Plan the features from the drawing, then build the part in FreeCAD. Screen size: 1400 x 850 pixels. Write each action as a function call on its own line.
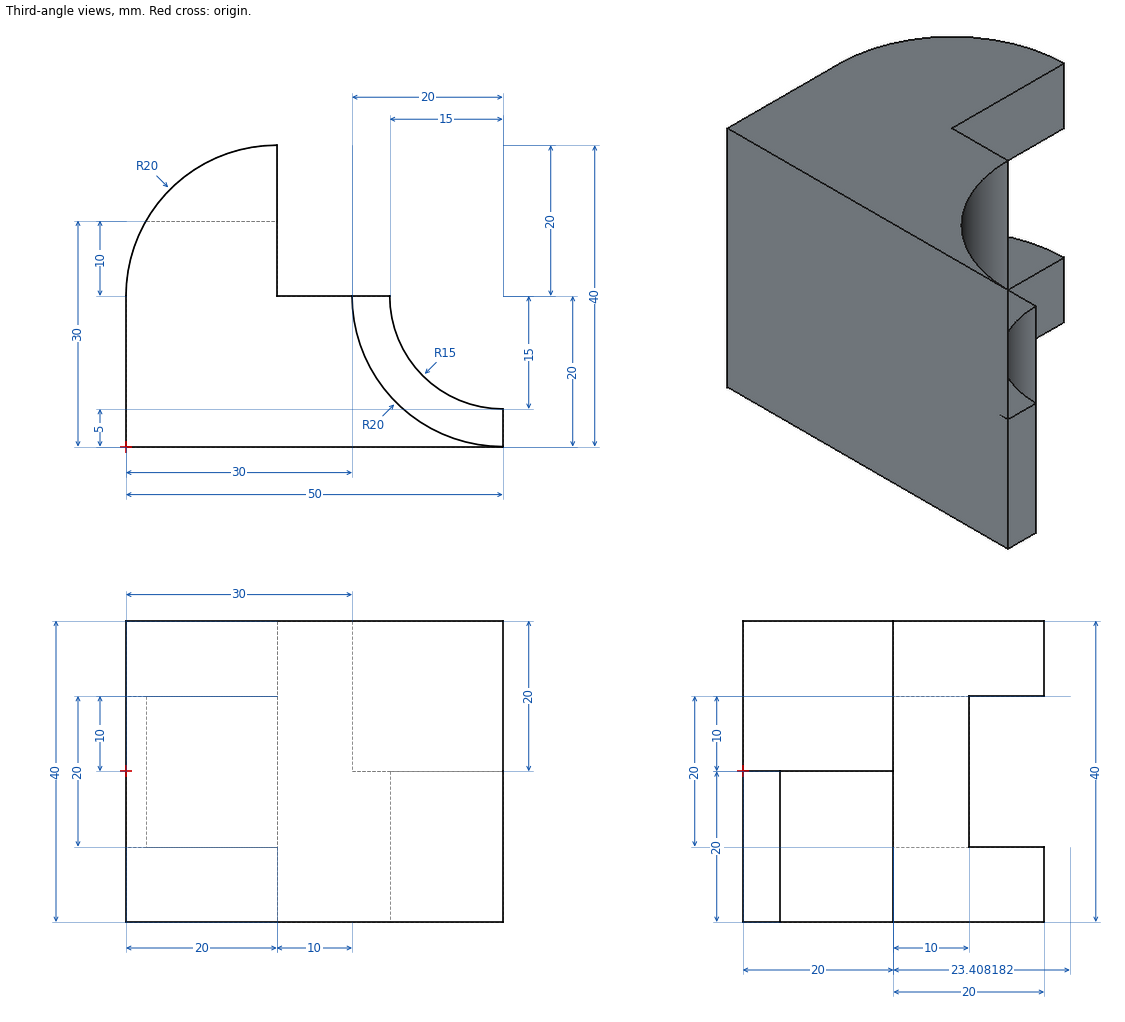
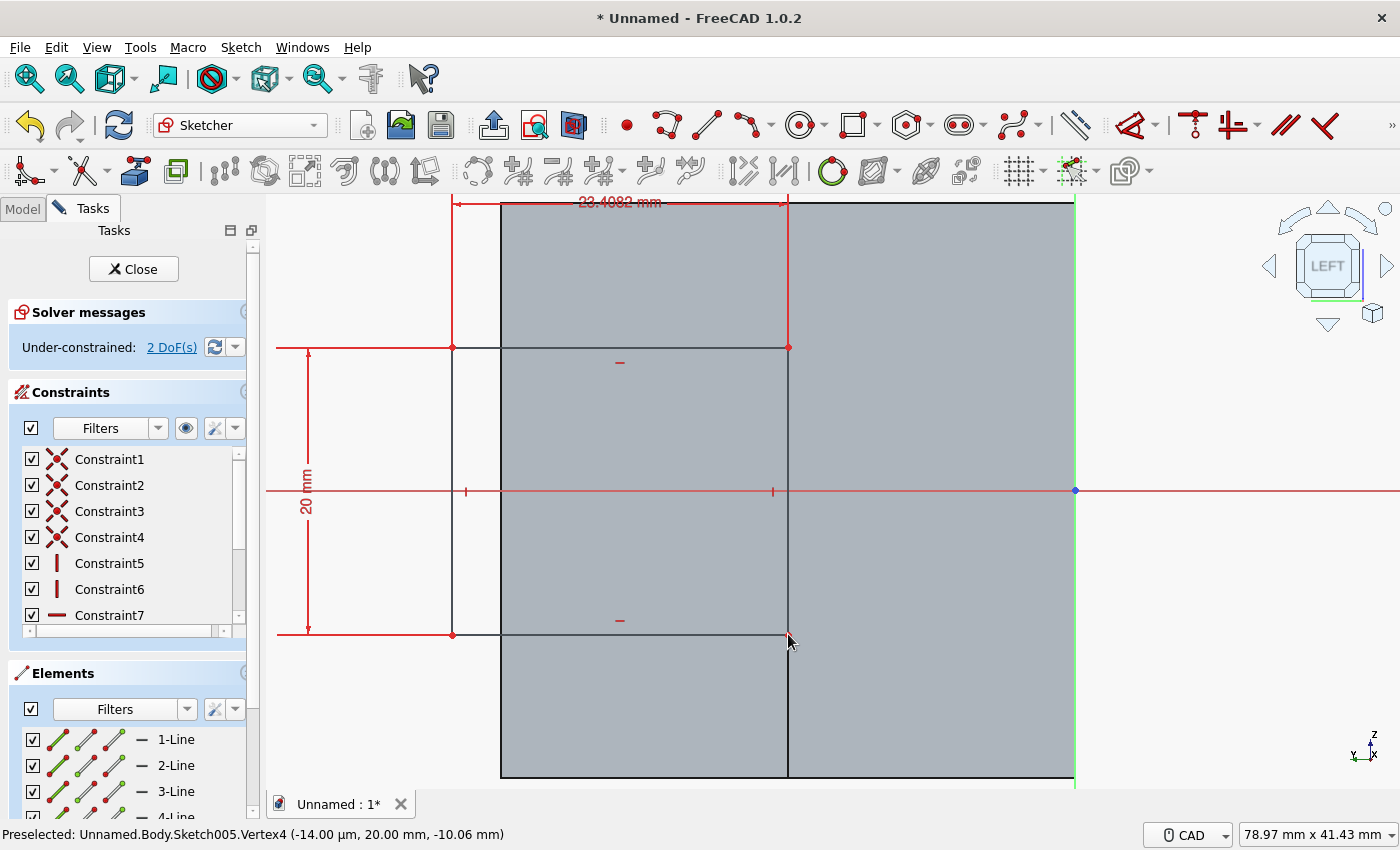
key(d)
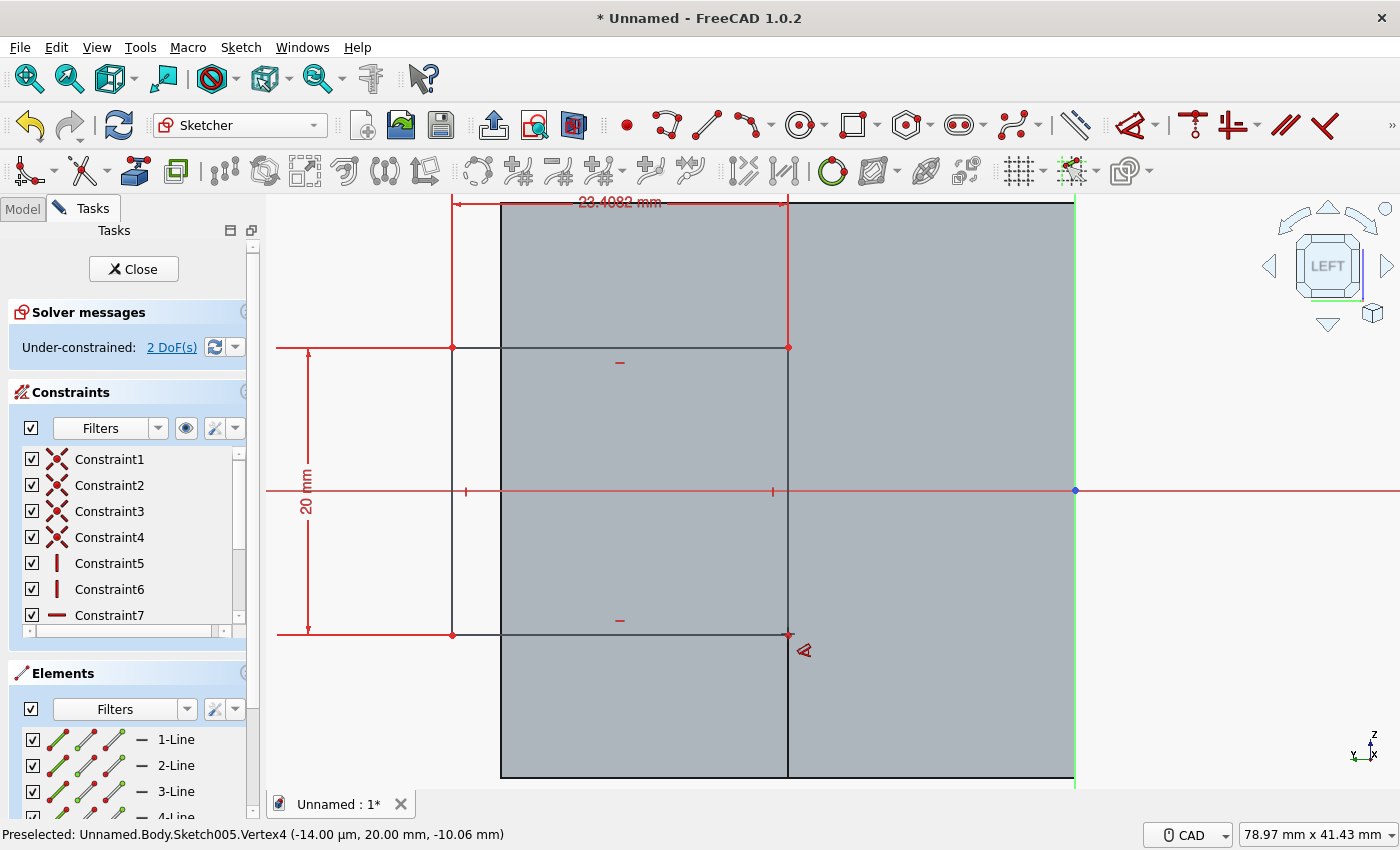
click(452, 348)
click(418, 419)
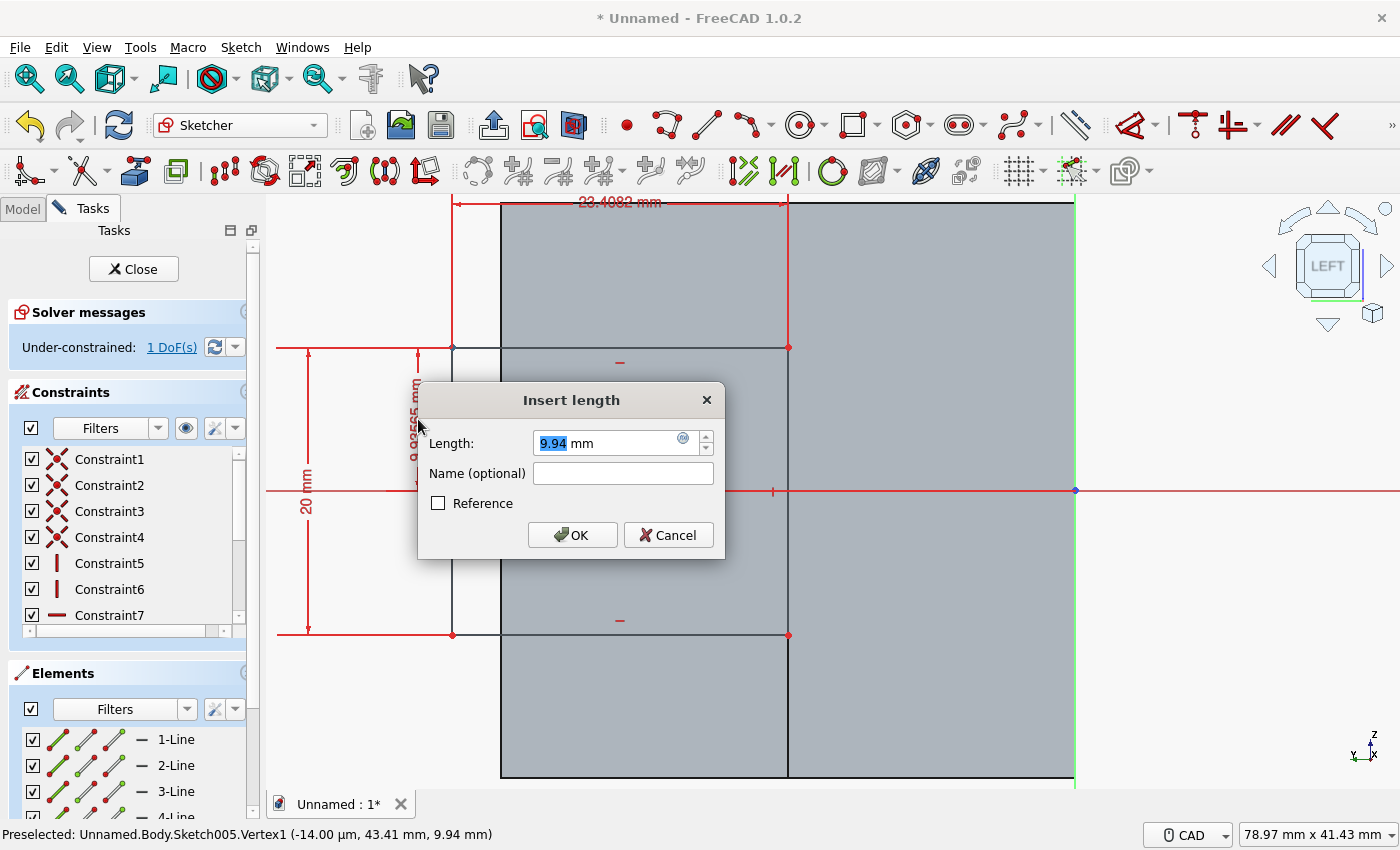
text(10)
key(Return)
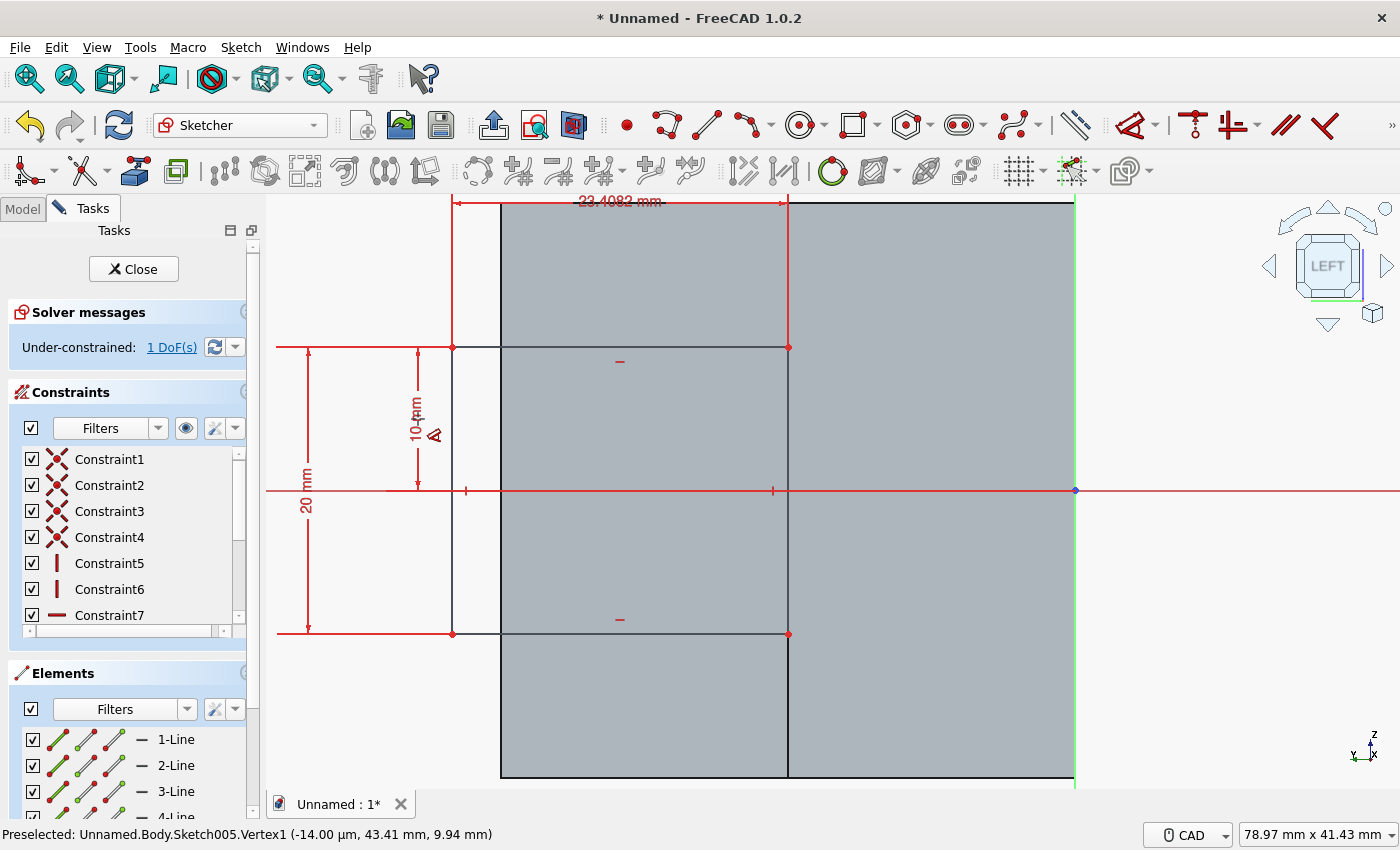
click(788, 634)
click(932, 668)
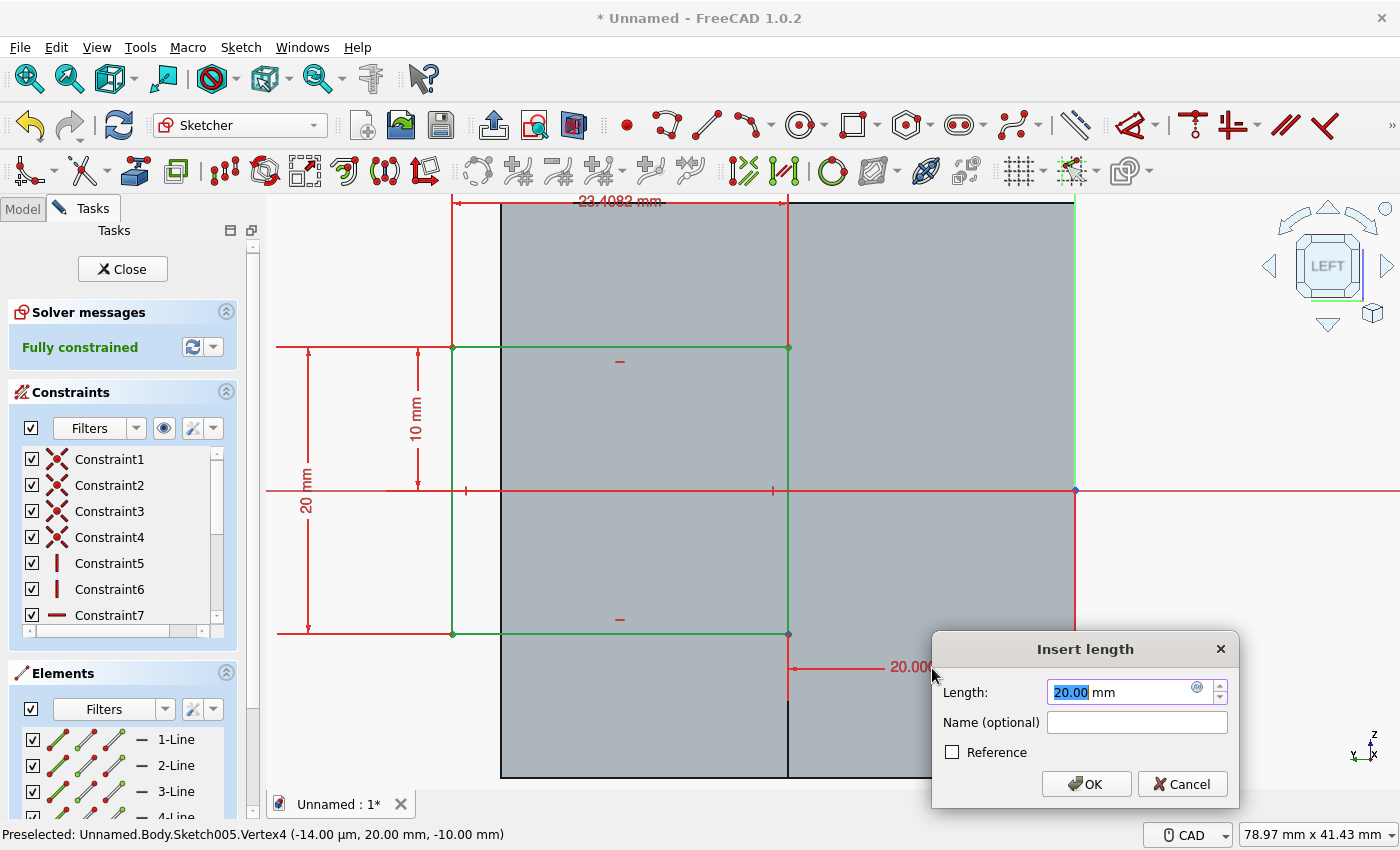
text(20)
key(Return)
key(Escape)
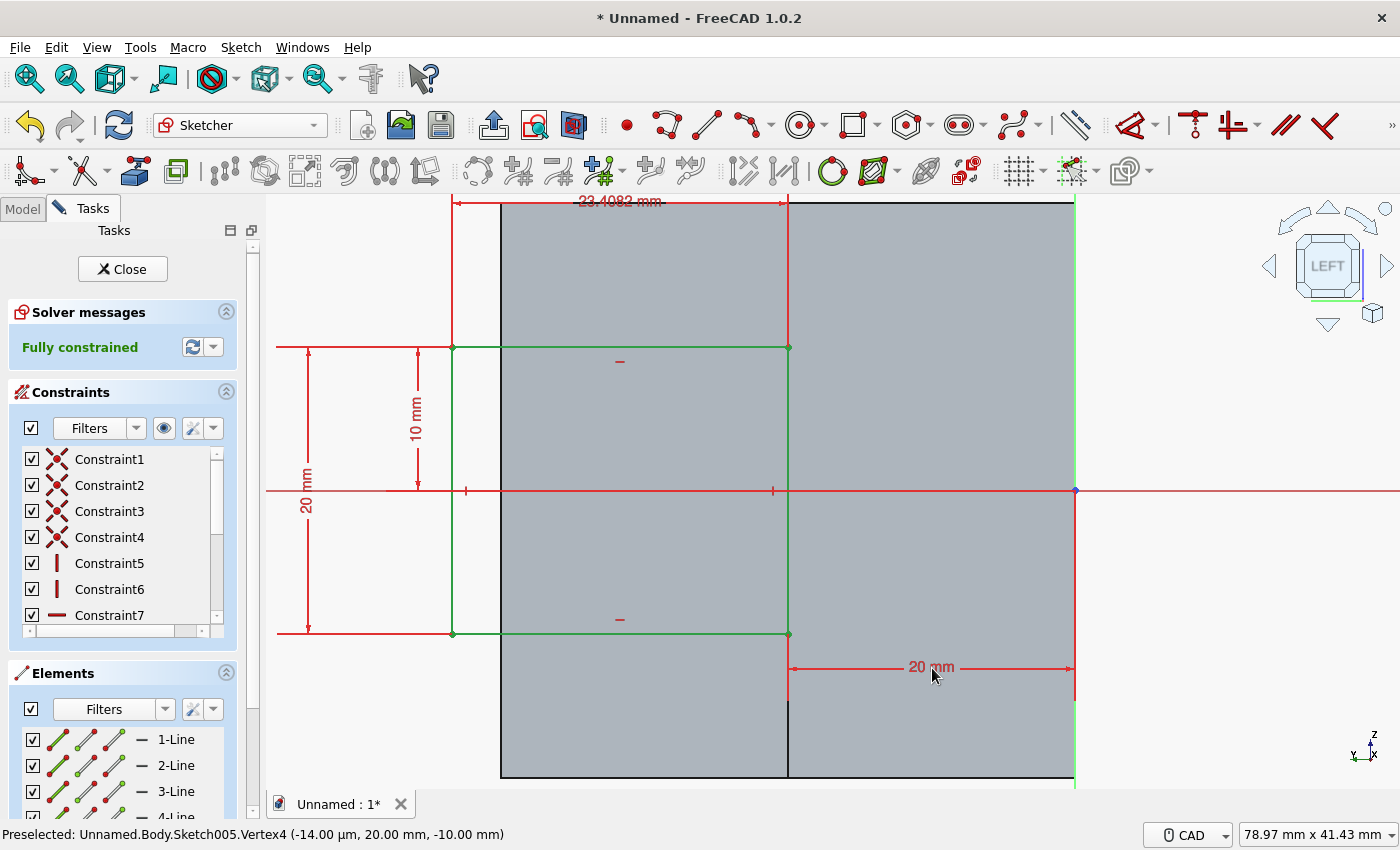
click(123, 269)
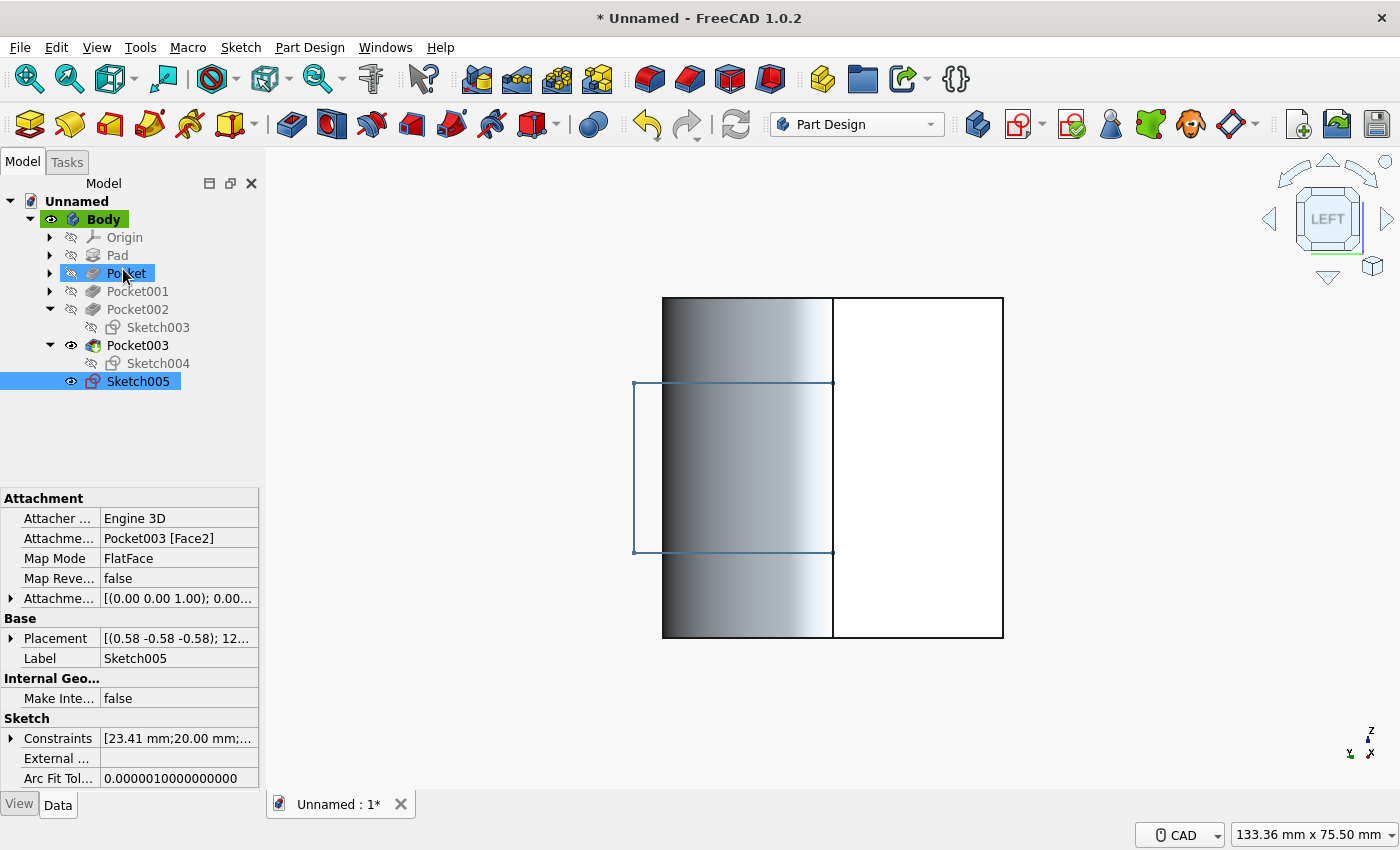
click(292, 124)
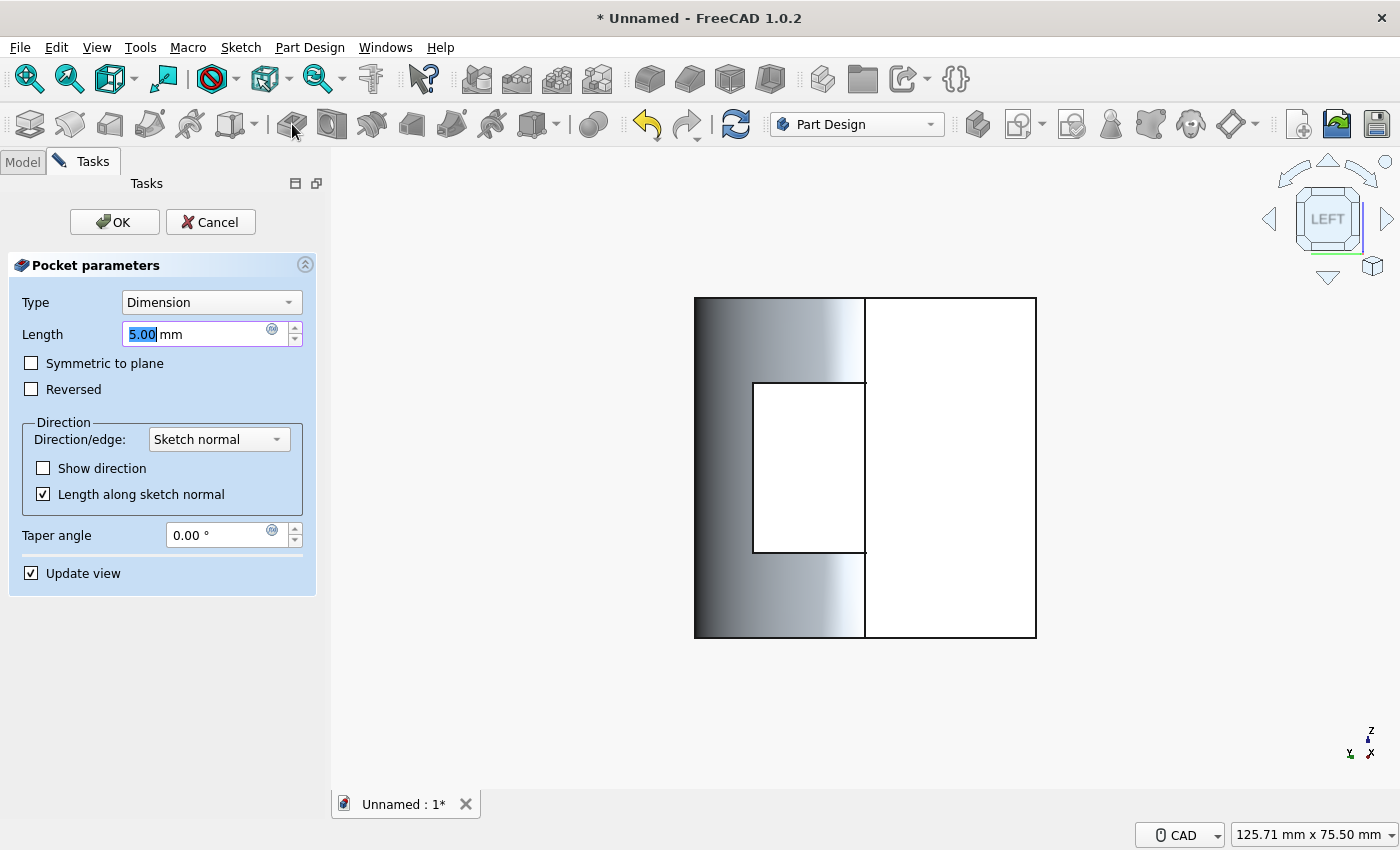
text(20)
key(Tab)